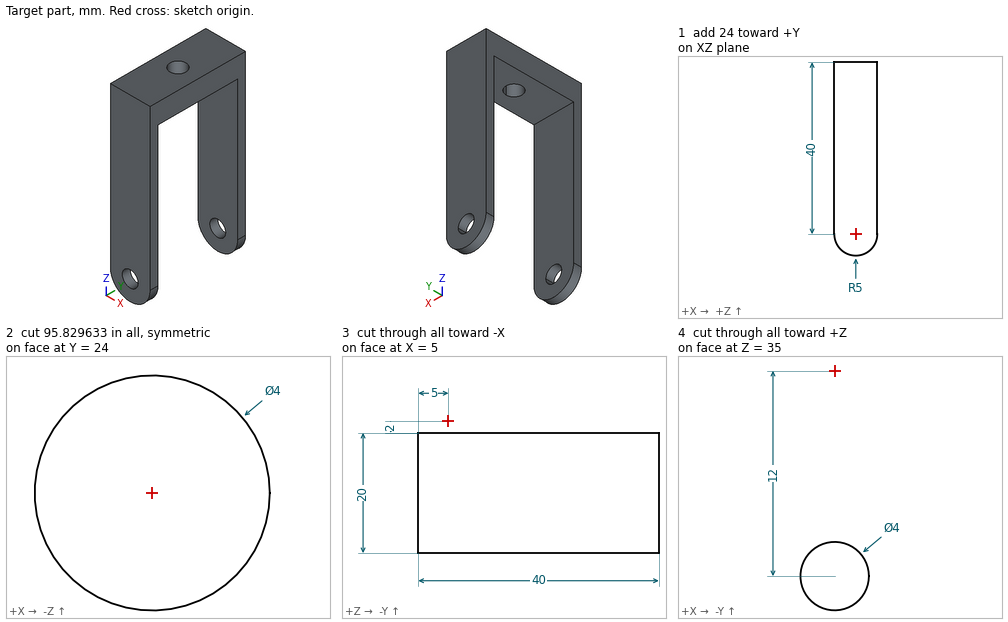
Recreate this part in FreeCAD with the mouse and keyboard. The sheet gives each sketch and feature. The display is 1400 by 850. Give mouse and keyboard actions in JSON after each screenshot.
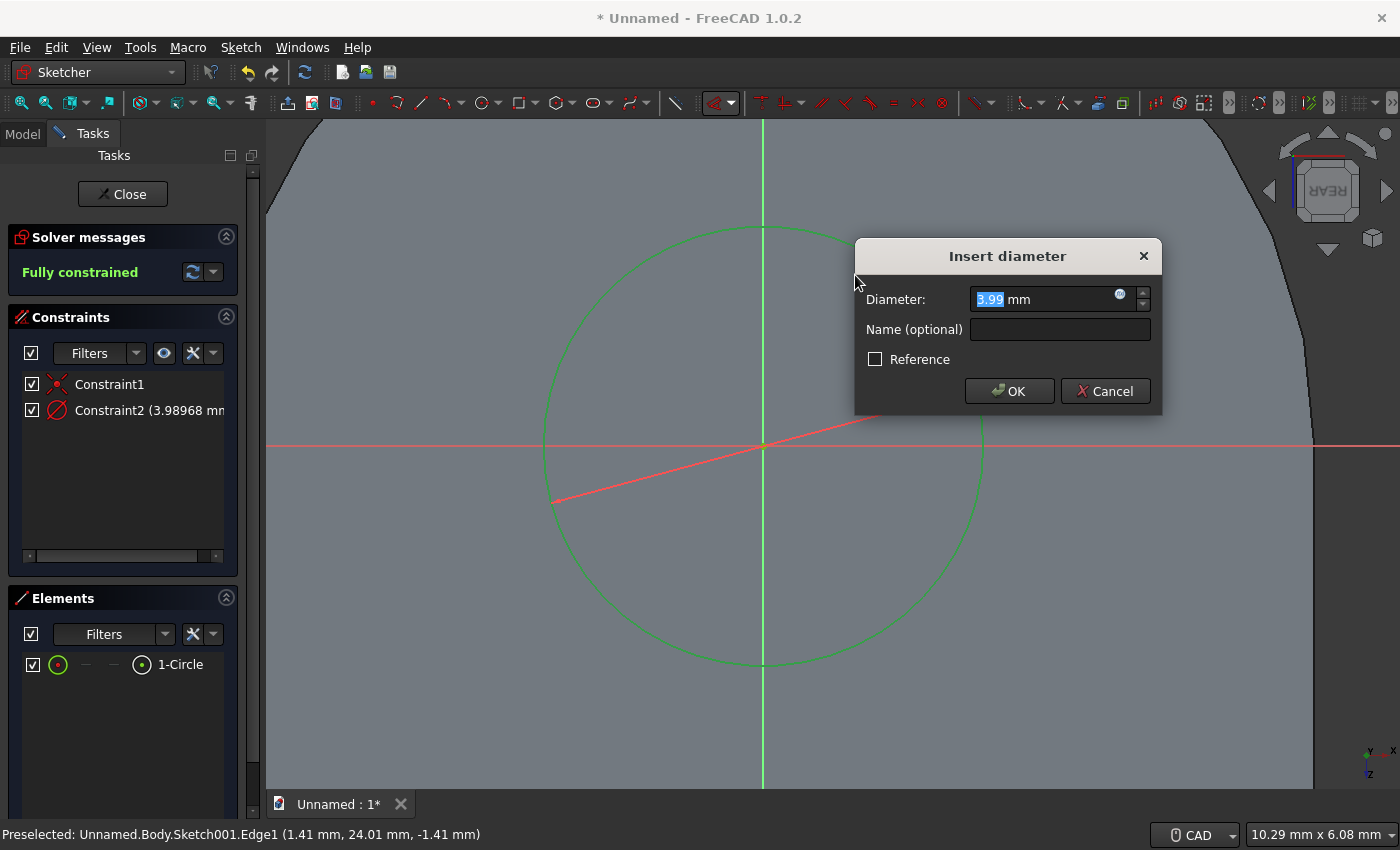
{"action": "type", "text": "4"}
{"action": "key", "text": "Return"}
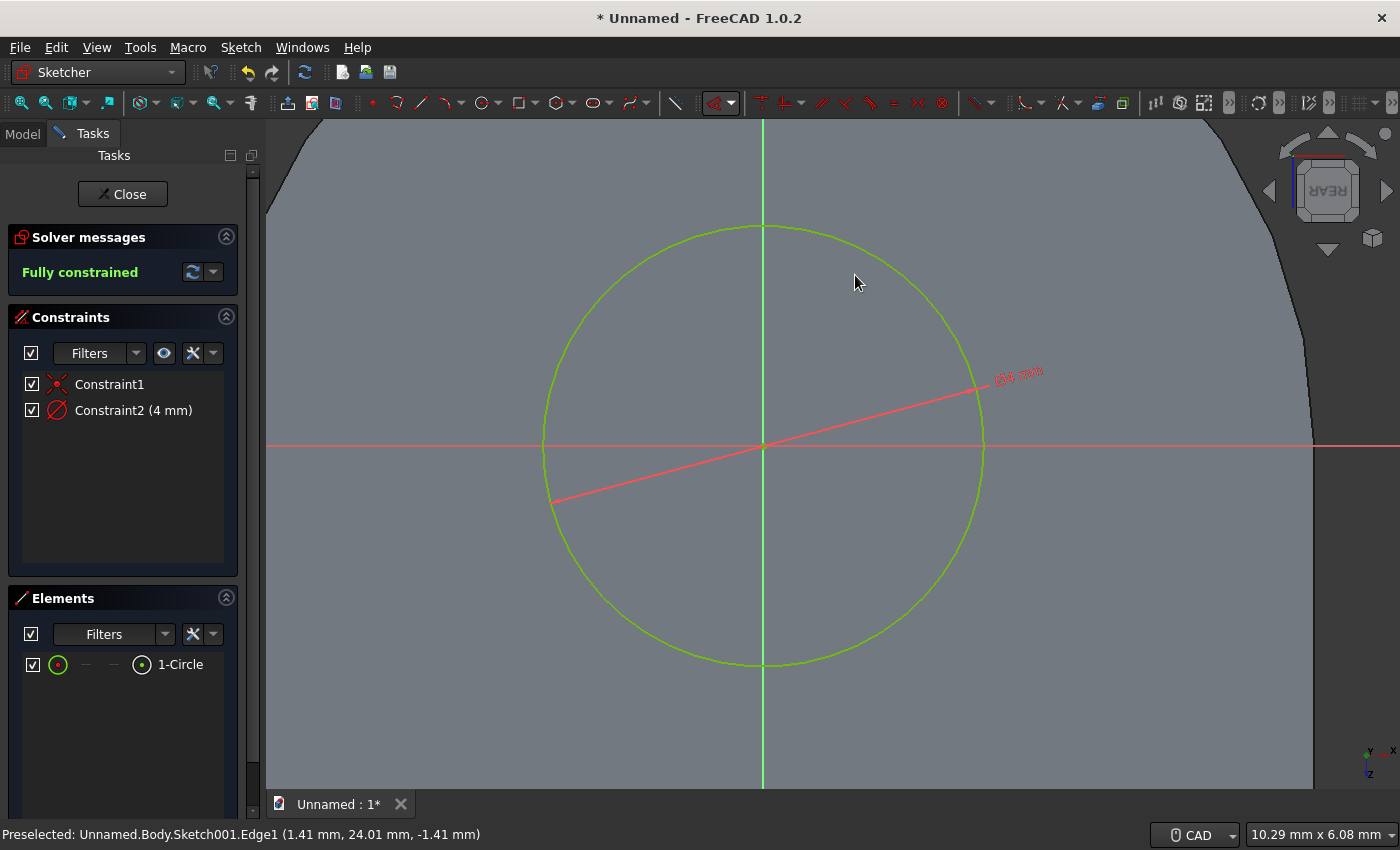
{"action": "left_click", "coordinate": [123, 194]}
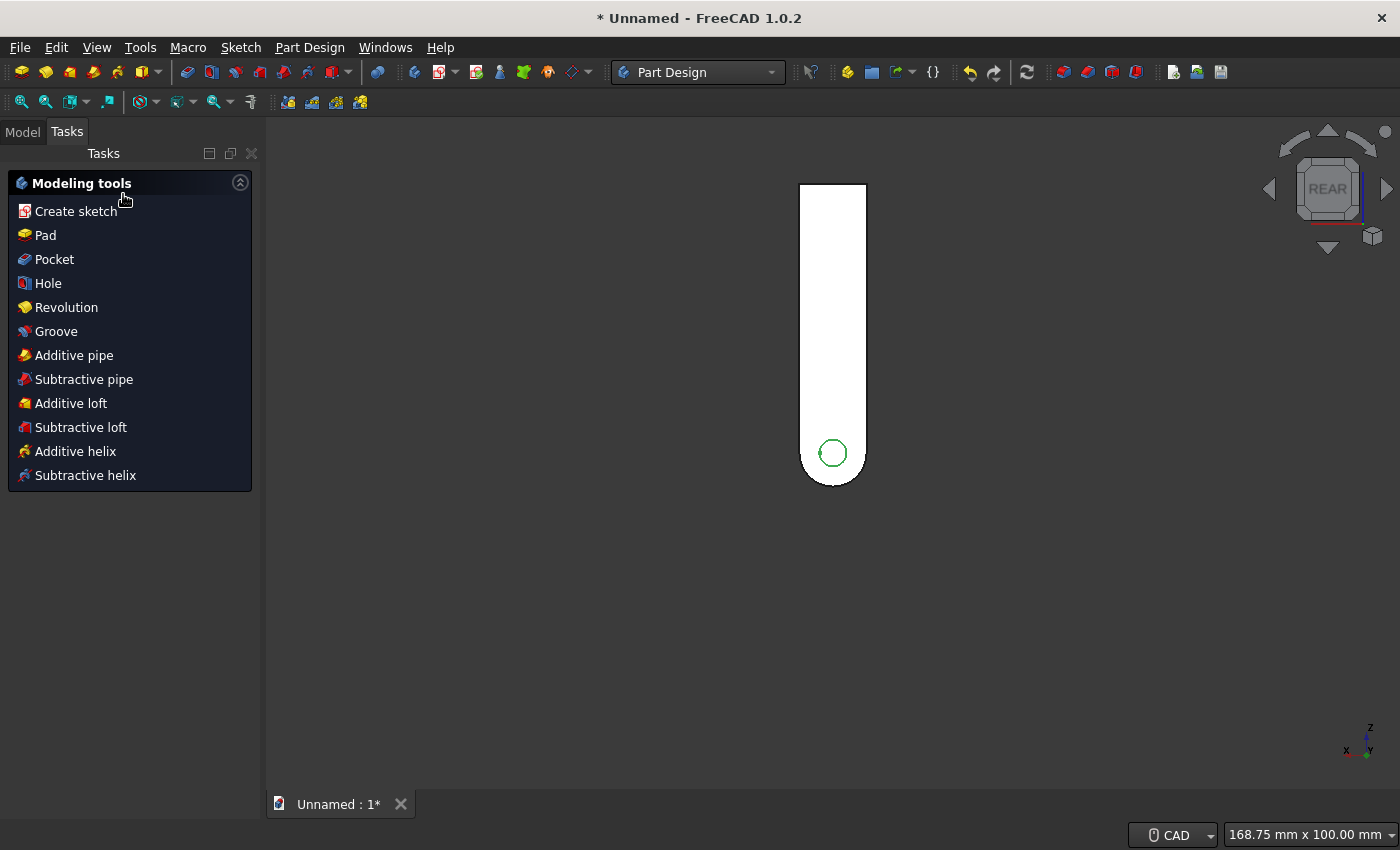
{"action": "left_click", "coordinate": [188, 72]}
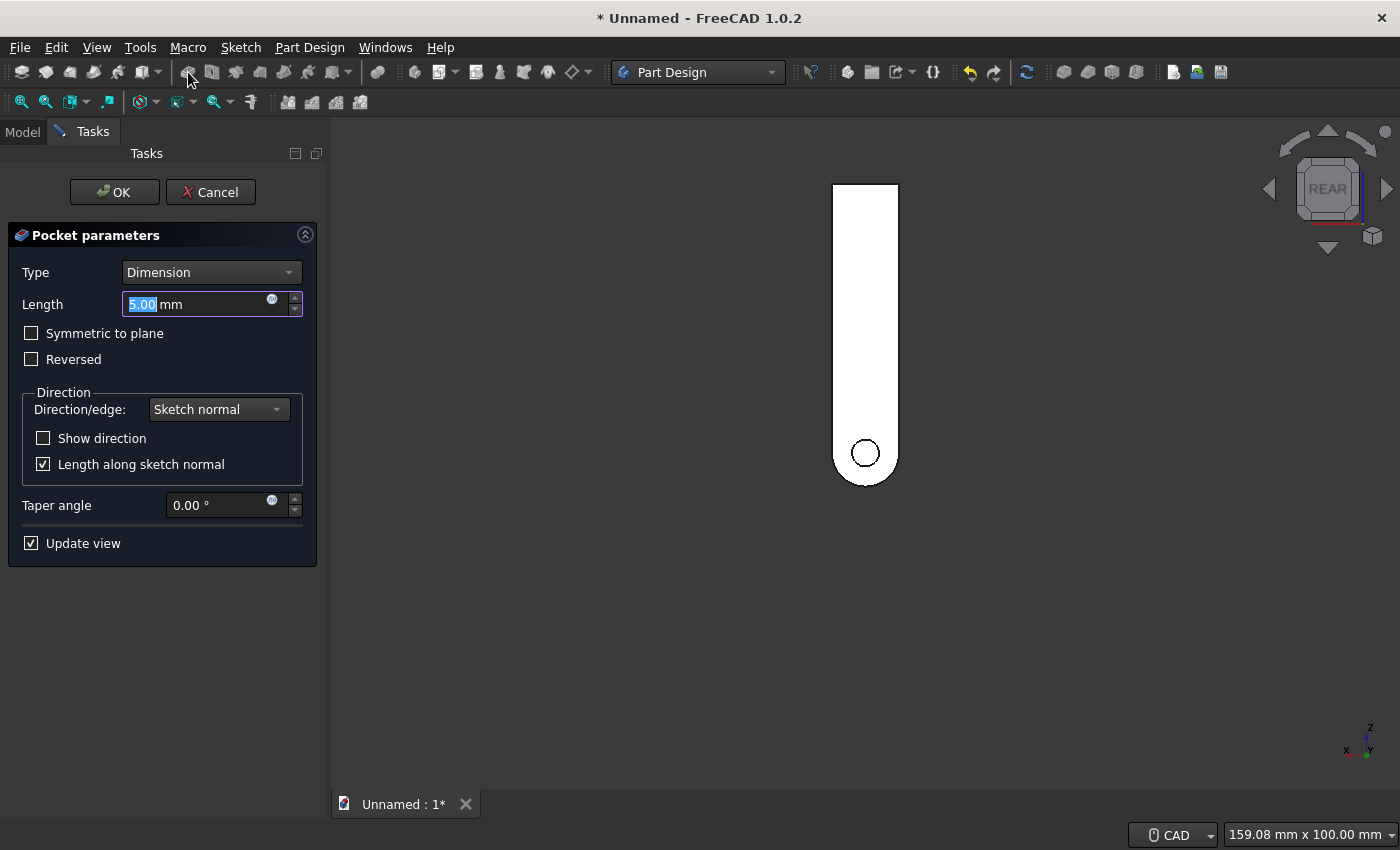
{"action": "type", "text": "95.829633"}
{"action": "key", "text": "Tab"}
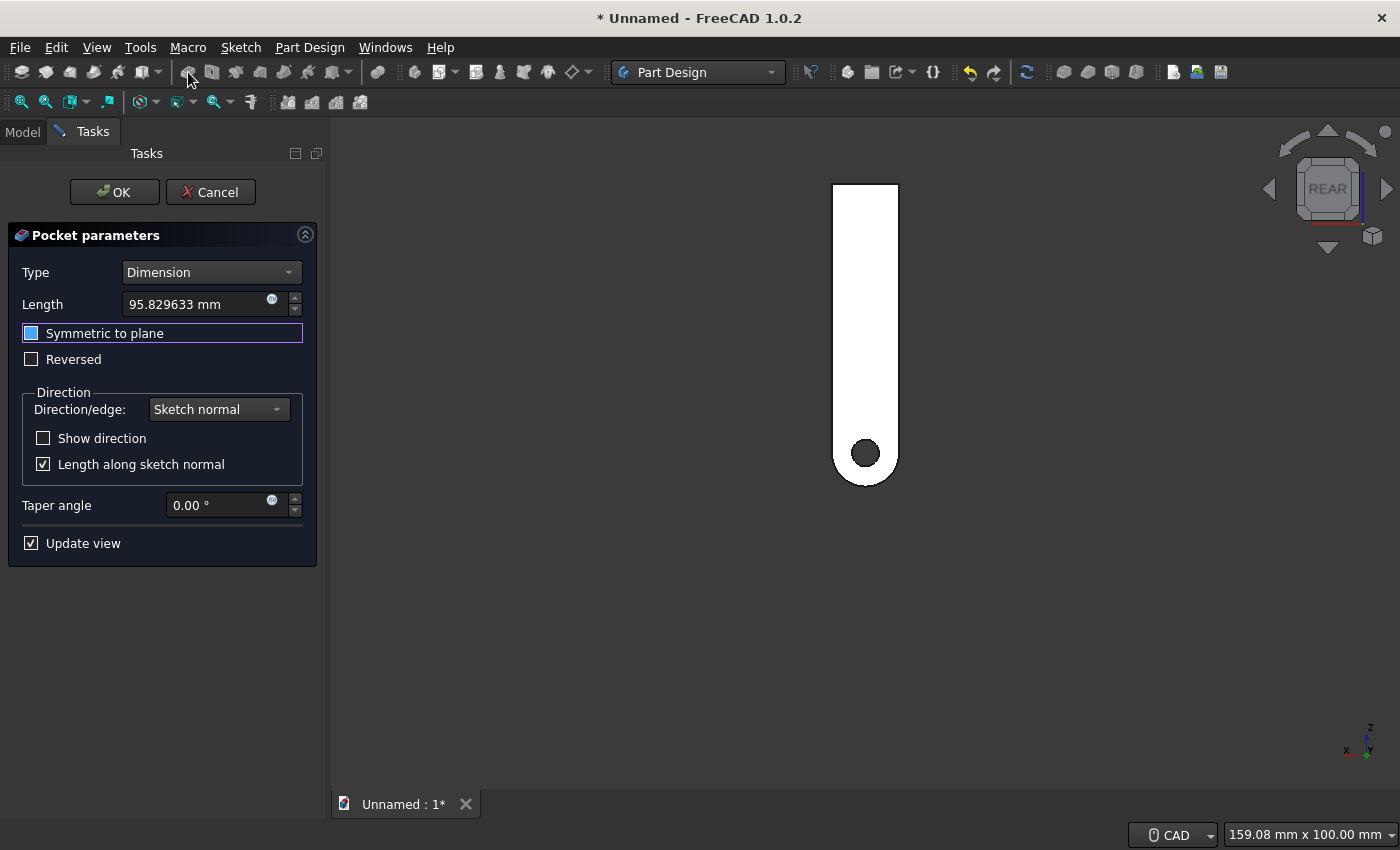
{"action": "left_click", "coordinate": [30, 333]}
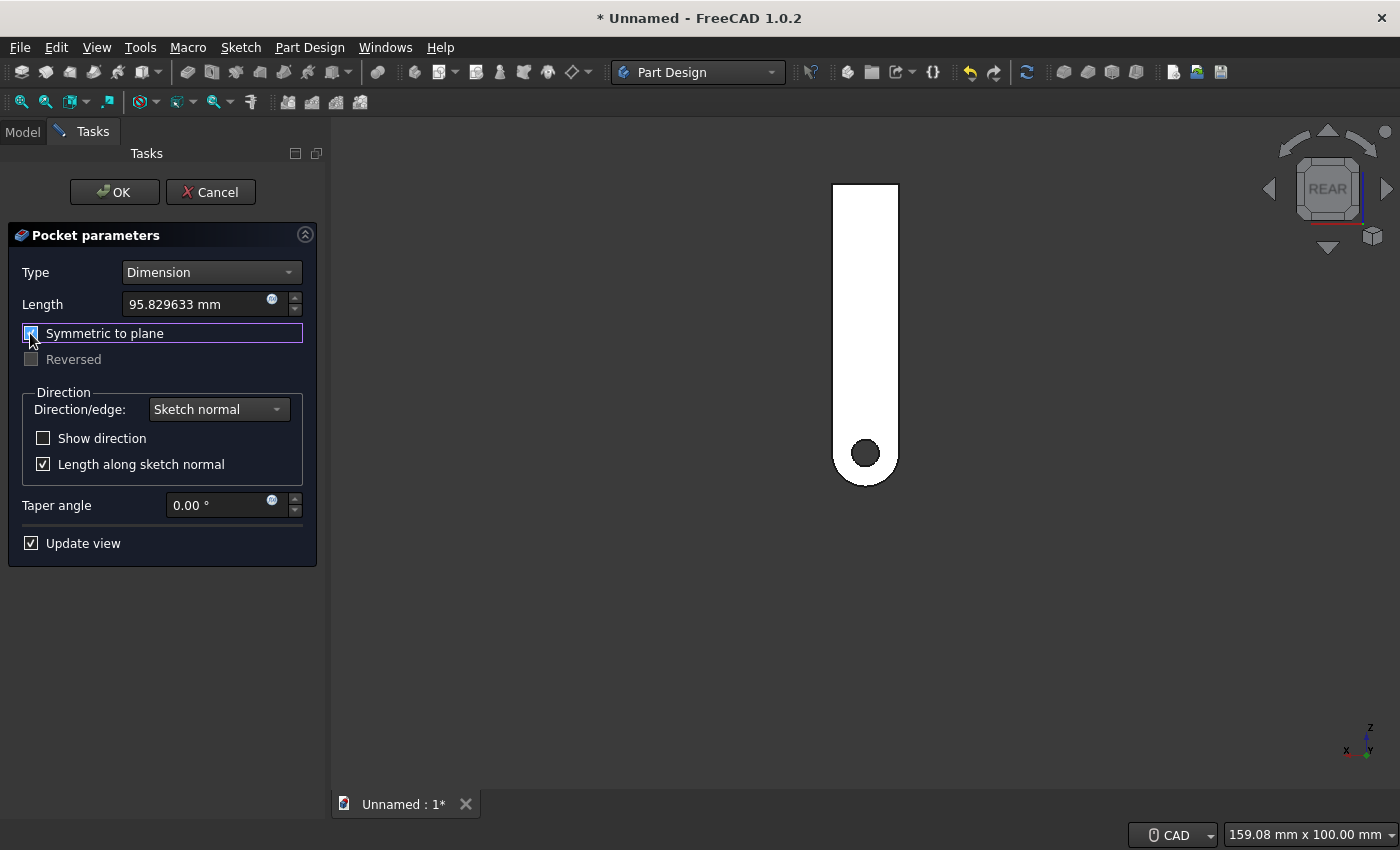
{"action": "left_click", "coordinate": [115, 192]}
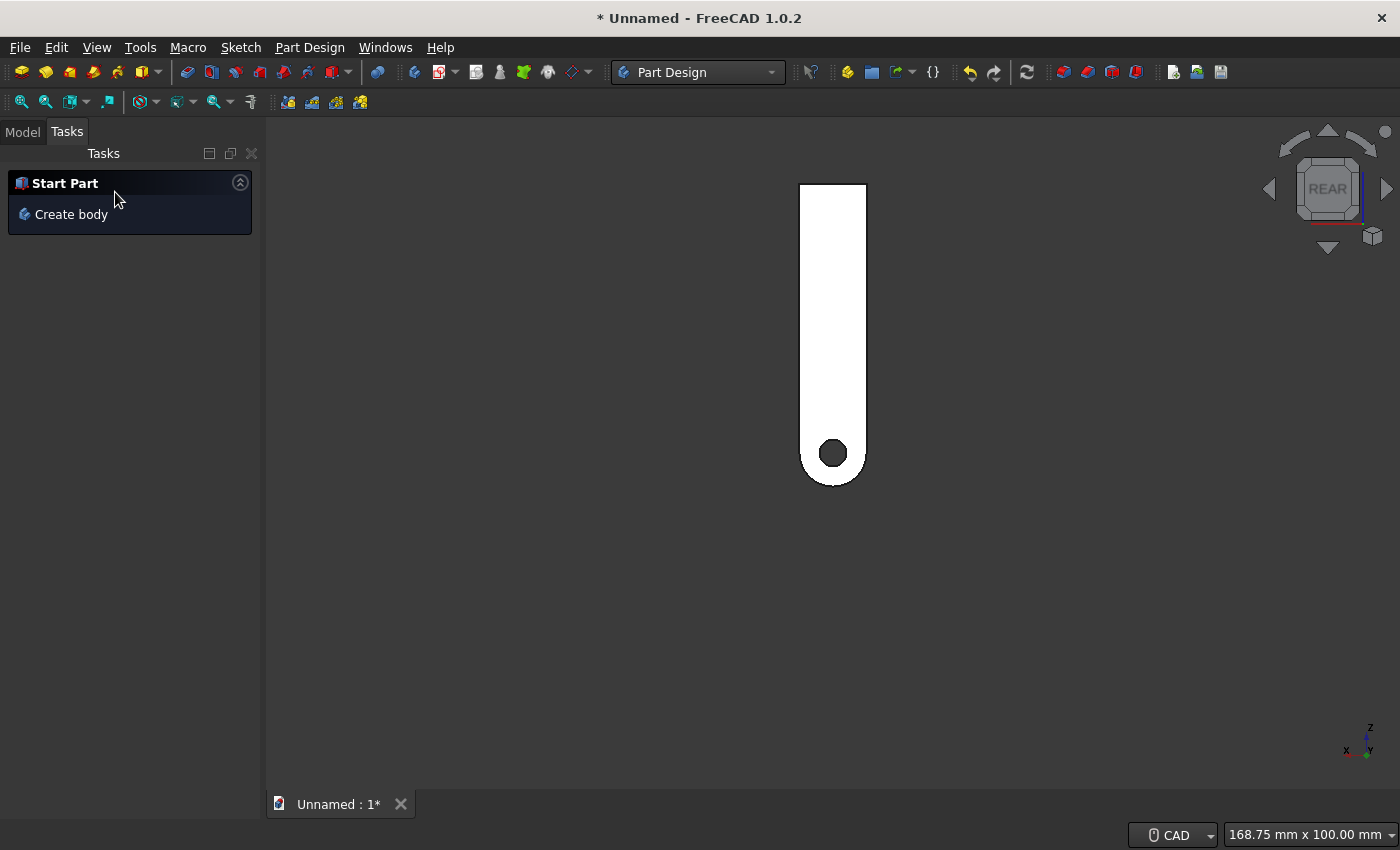
{"action": "key", "text": "0"}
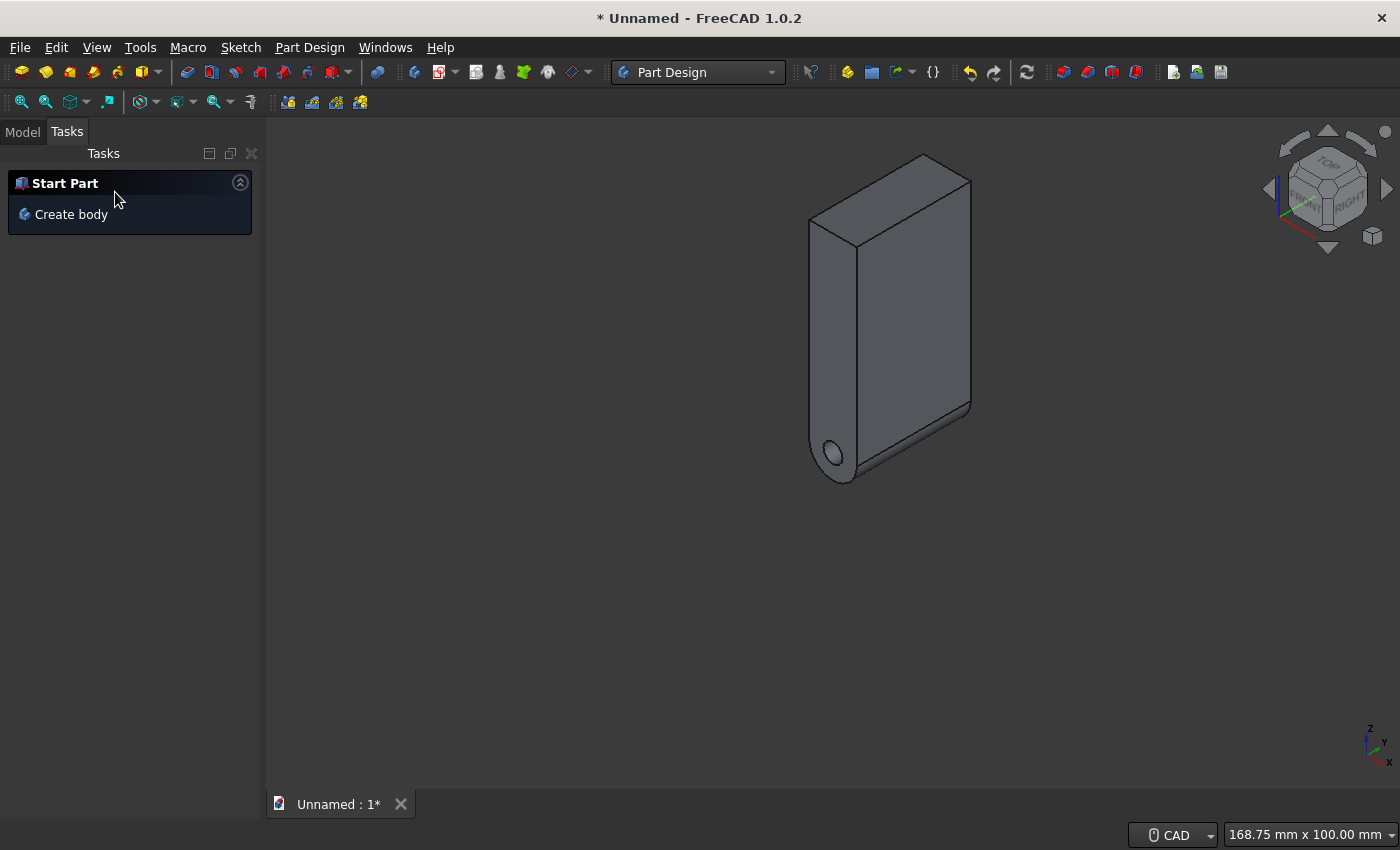
{"action": "left_click", "coordinate": [914, 292]}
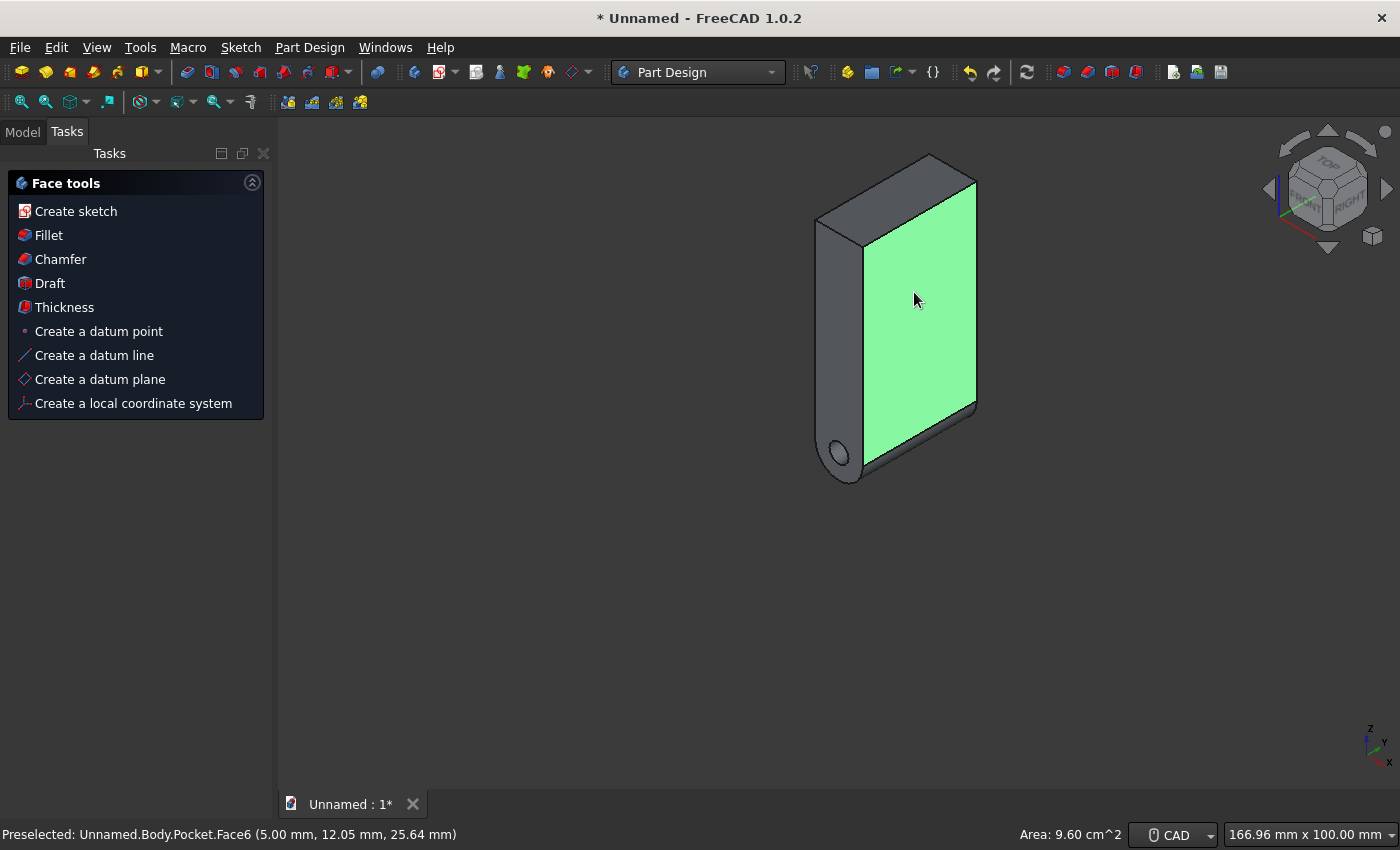
{"action": "left_click", "coordinate": [440, 72]}